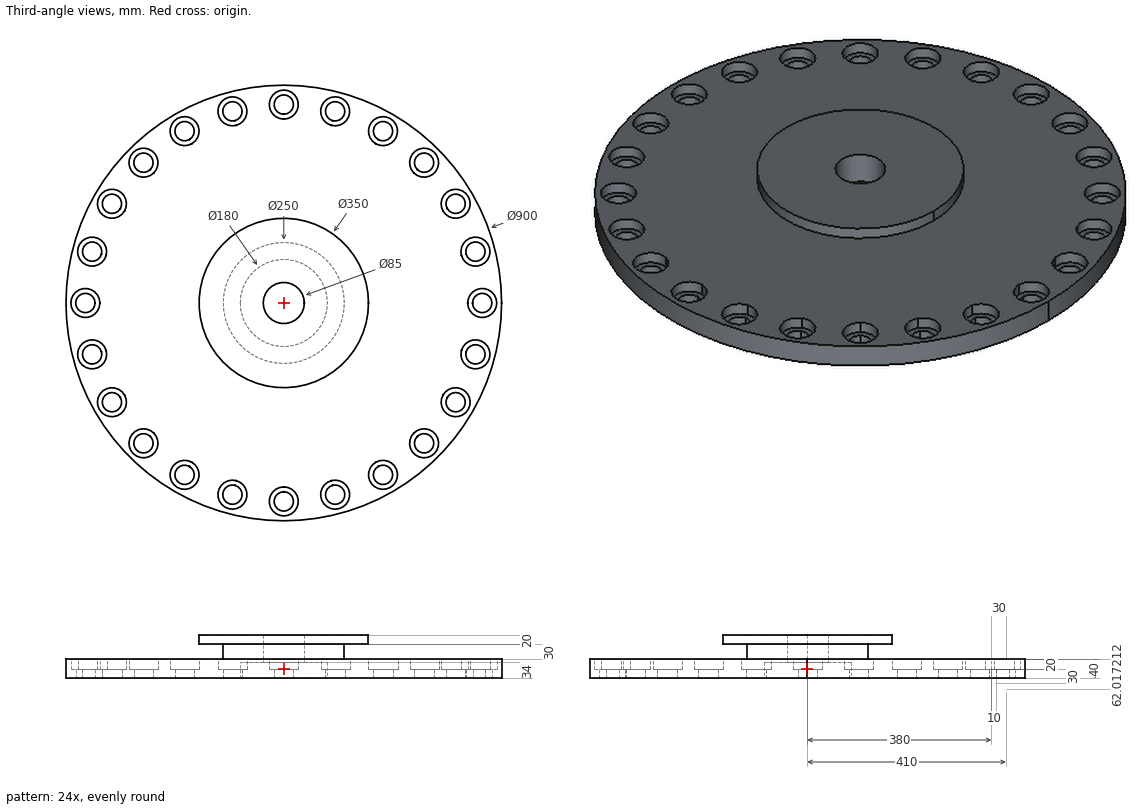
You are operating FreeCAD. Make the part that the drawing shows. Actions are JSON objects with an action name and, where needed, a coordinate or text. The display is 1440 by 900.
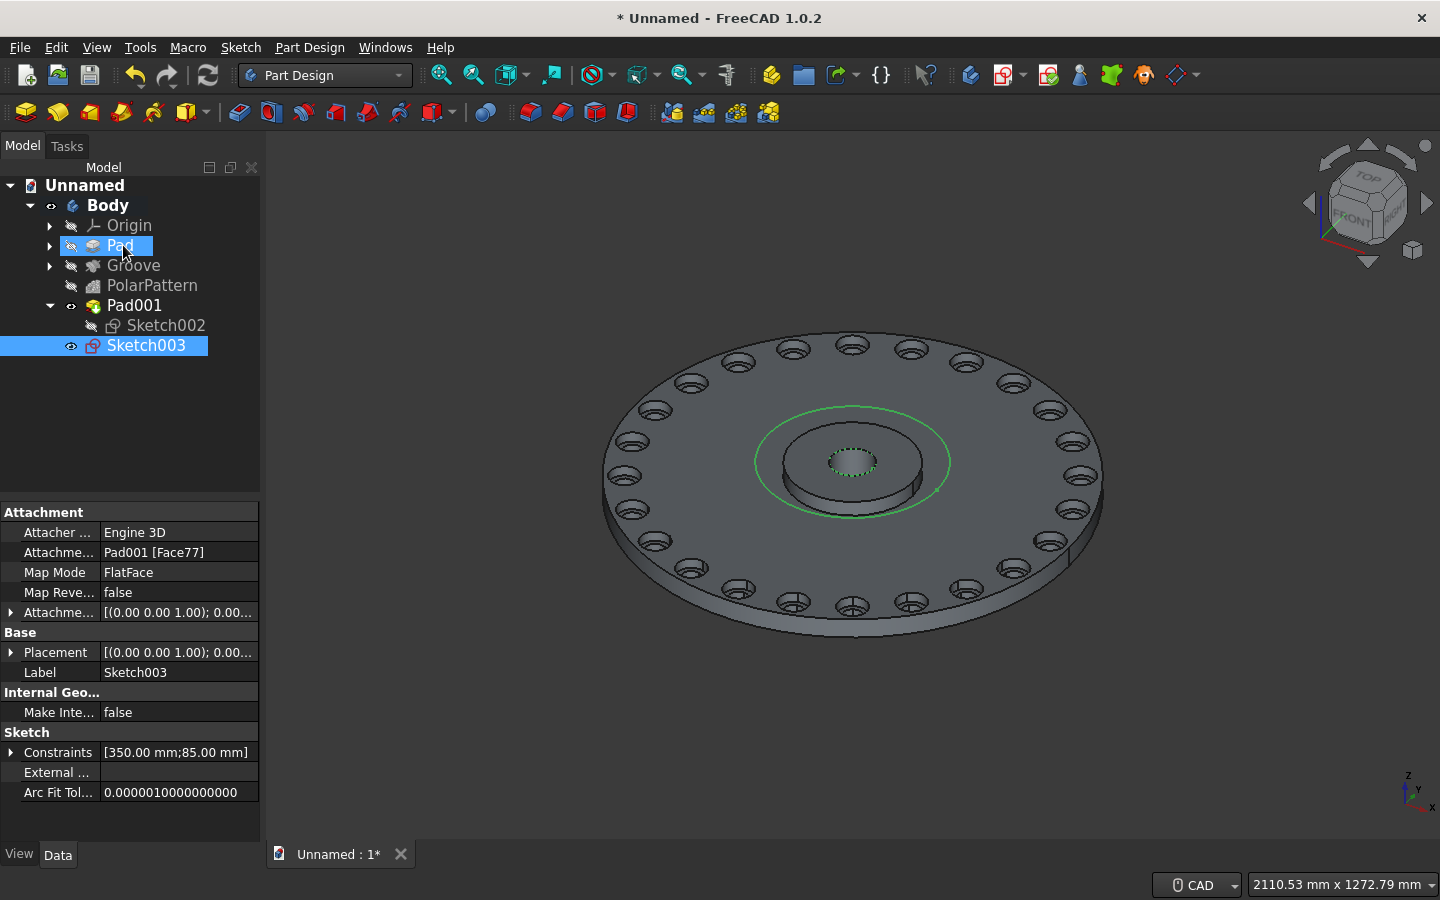
{"action": "left_click", "coordinate": [26, 112]}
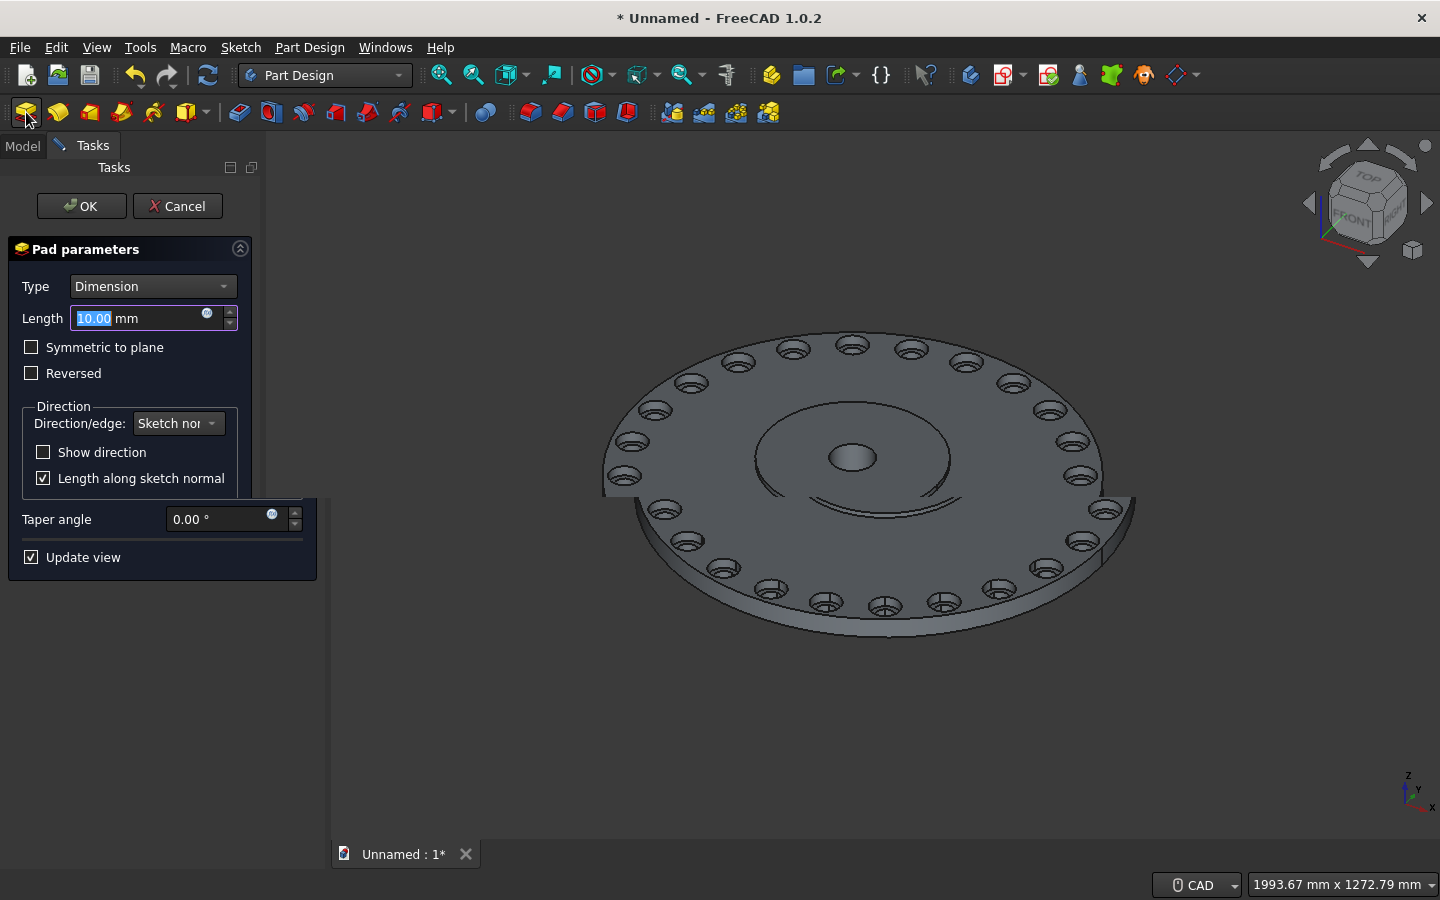
{"action": "type", "text": "20"}
{"action": "key", "text": "Tab"}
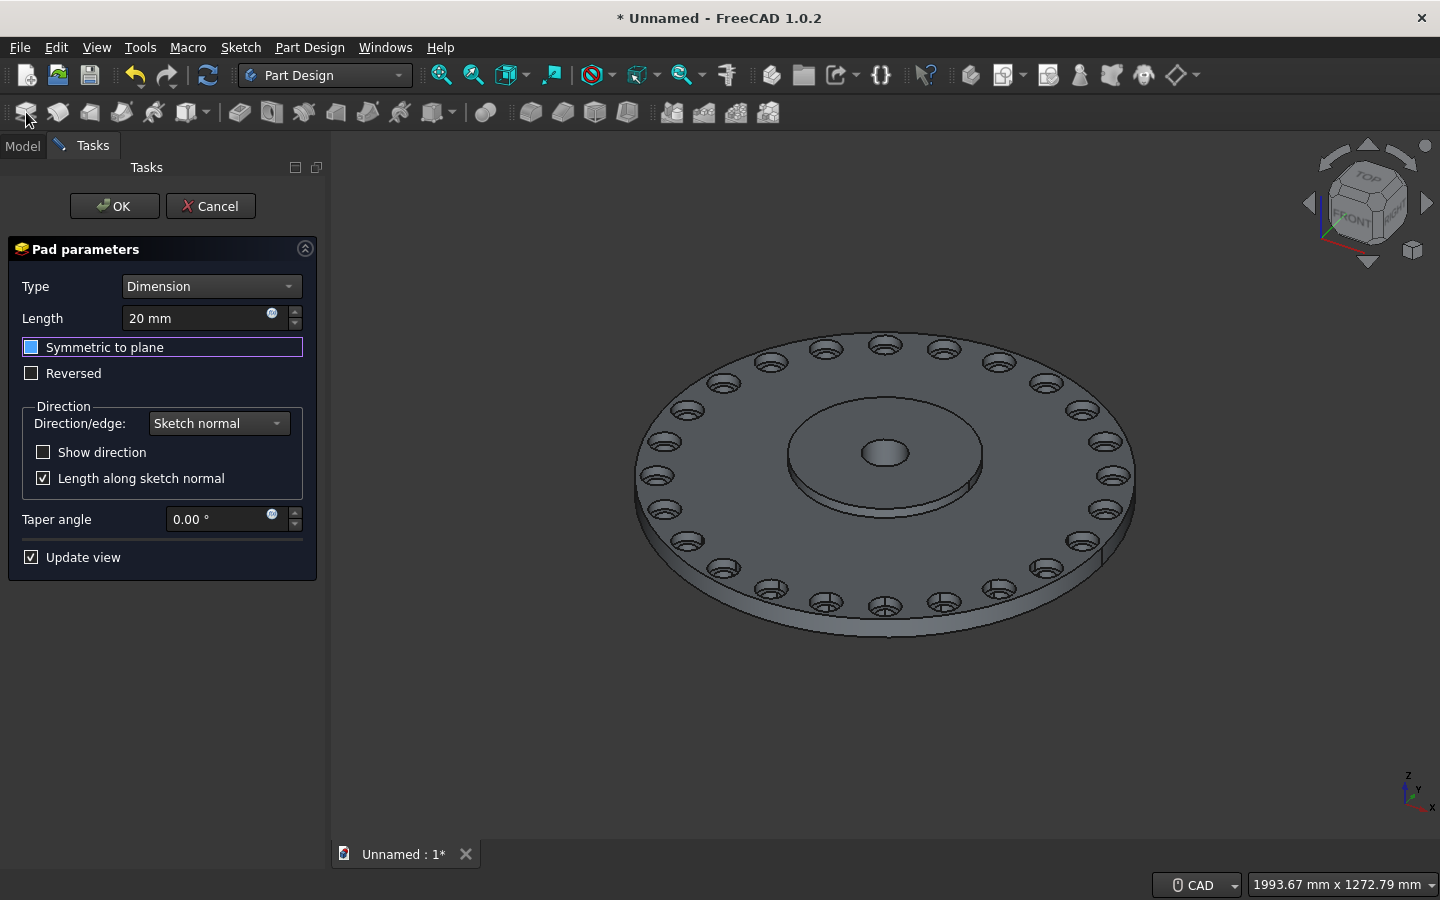
{"action": "left_click", "coordinate": [115, 206]}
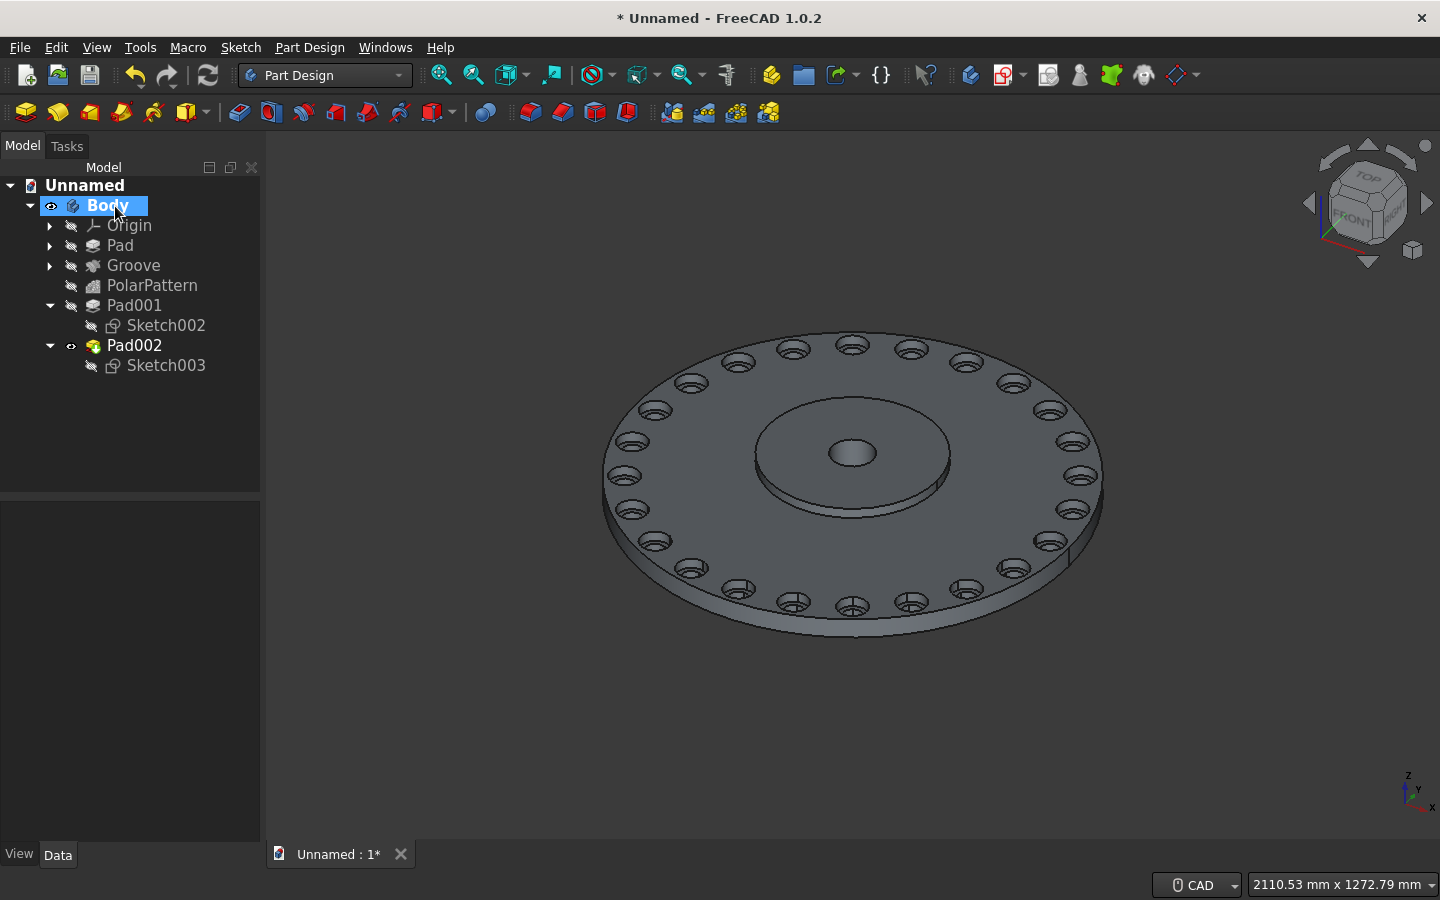
{"action": "key", "text": "5"}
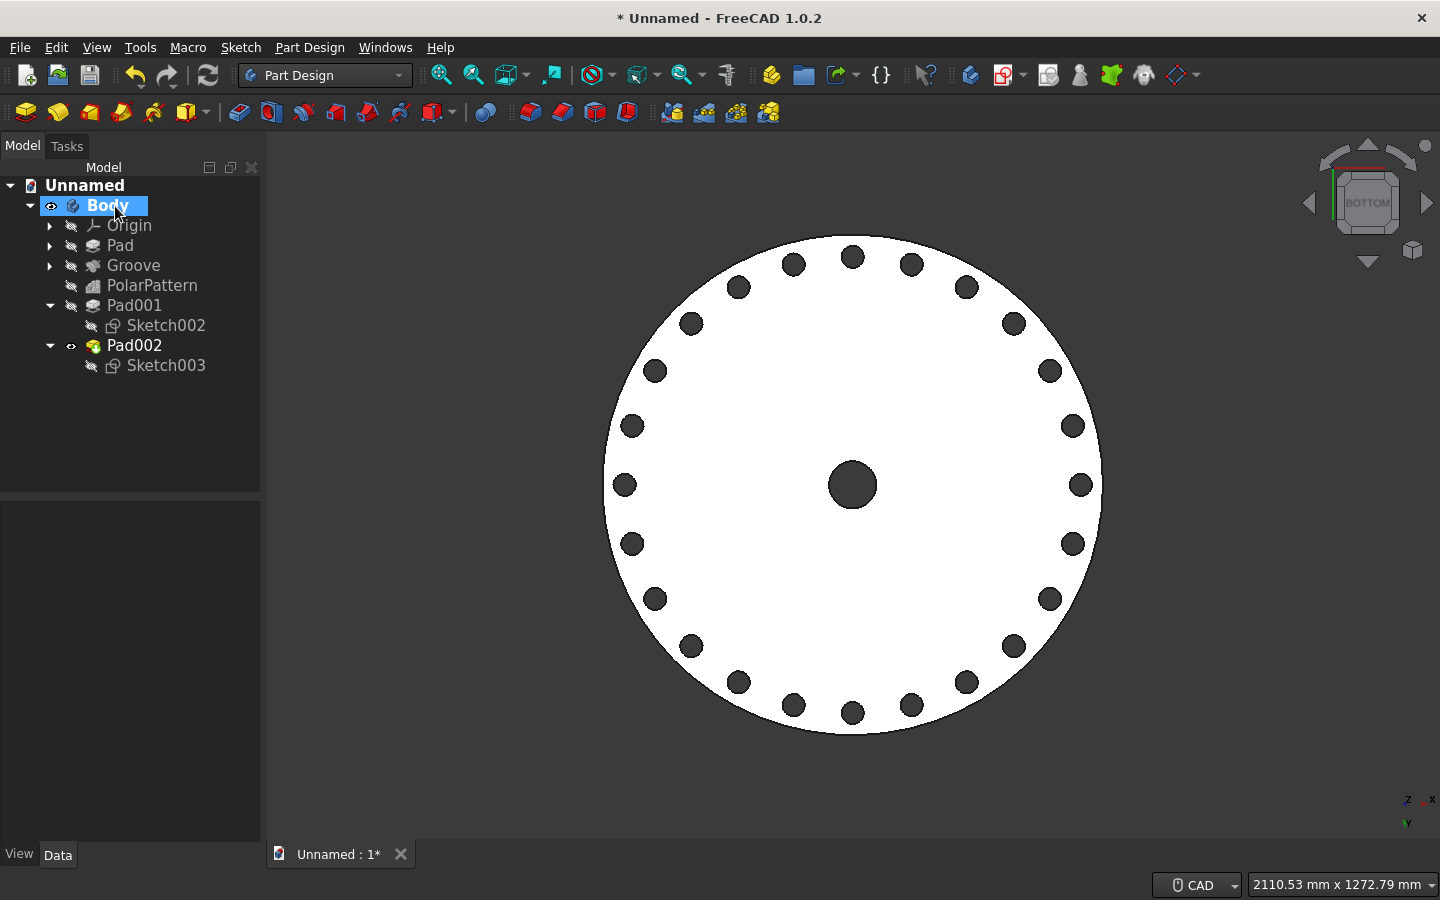
{"action": "left_click", "coordinate": [781, 412]}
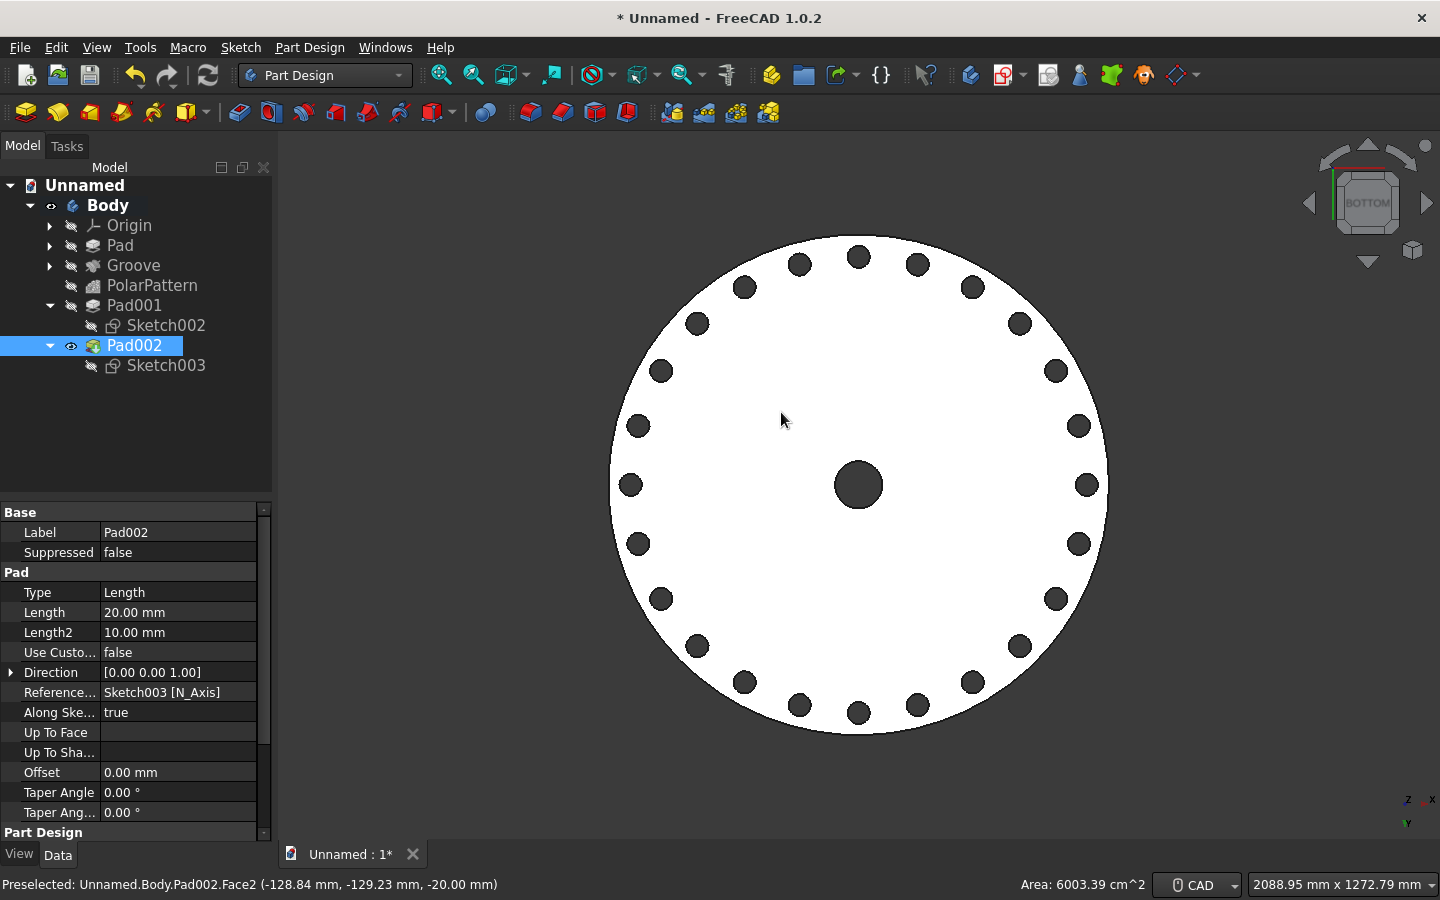
{"action": "left_click", "coordinate": [1004, 76]}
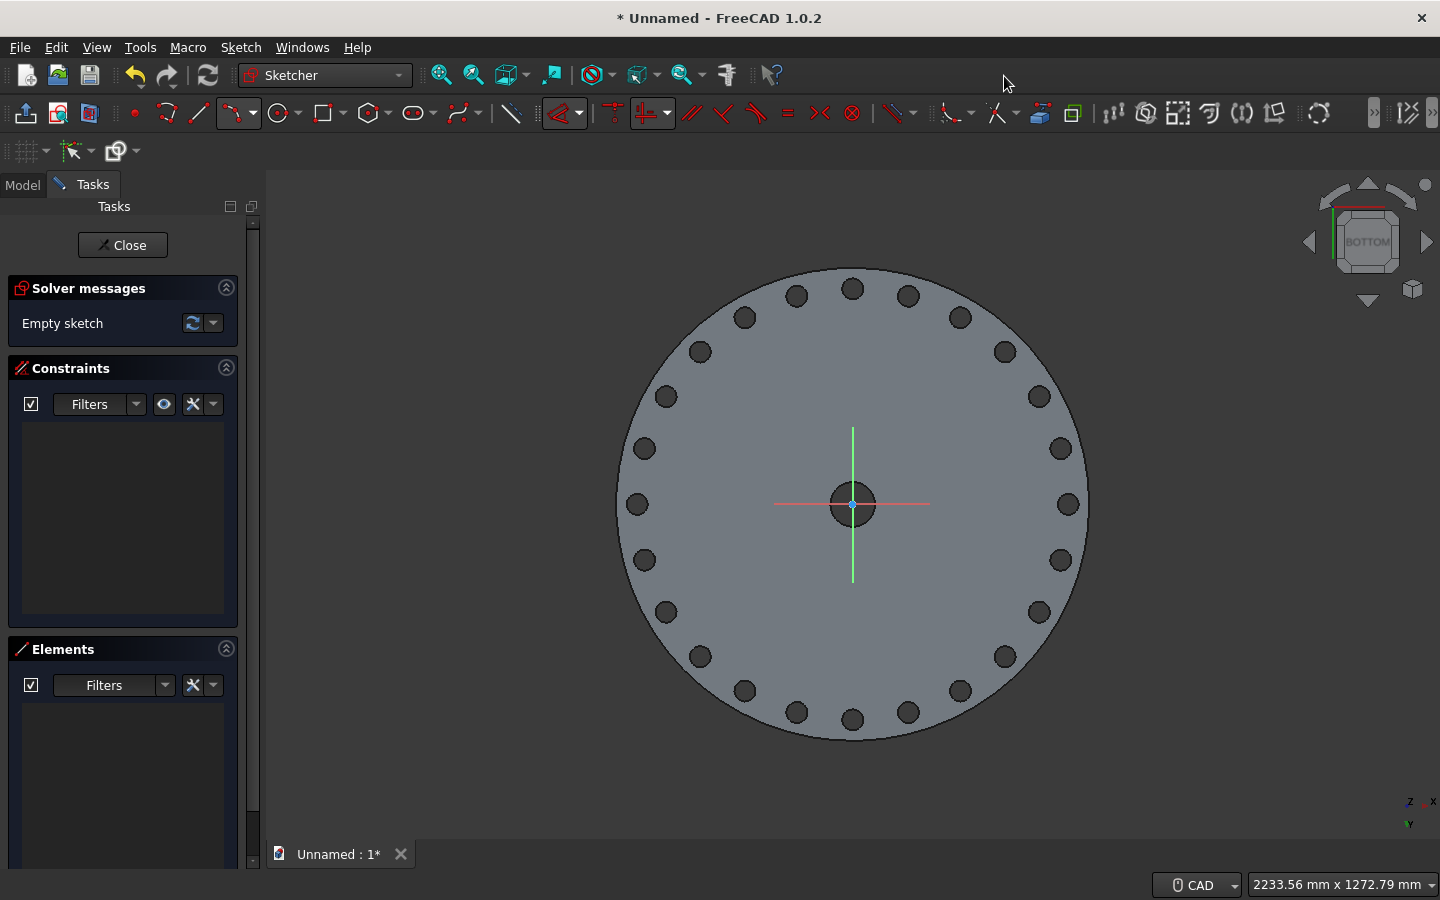
{"action": "scroll", "coordinate": [870, 504], "scroll_direction": "up", "scroll_amount": 8}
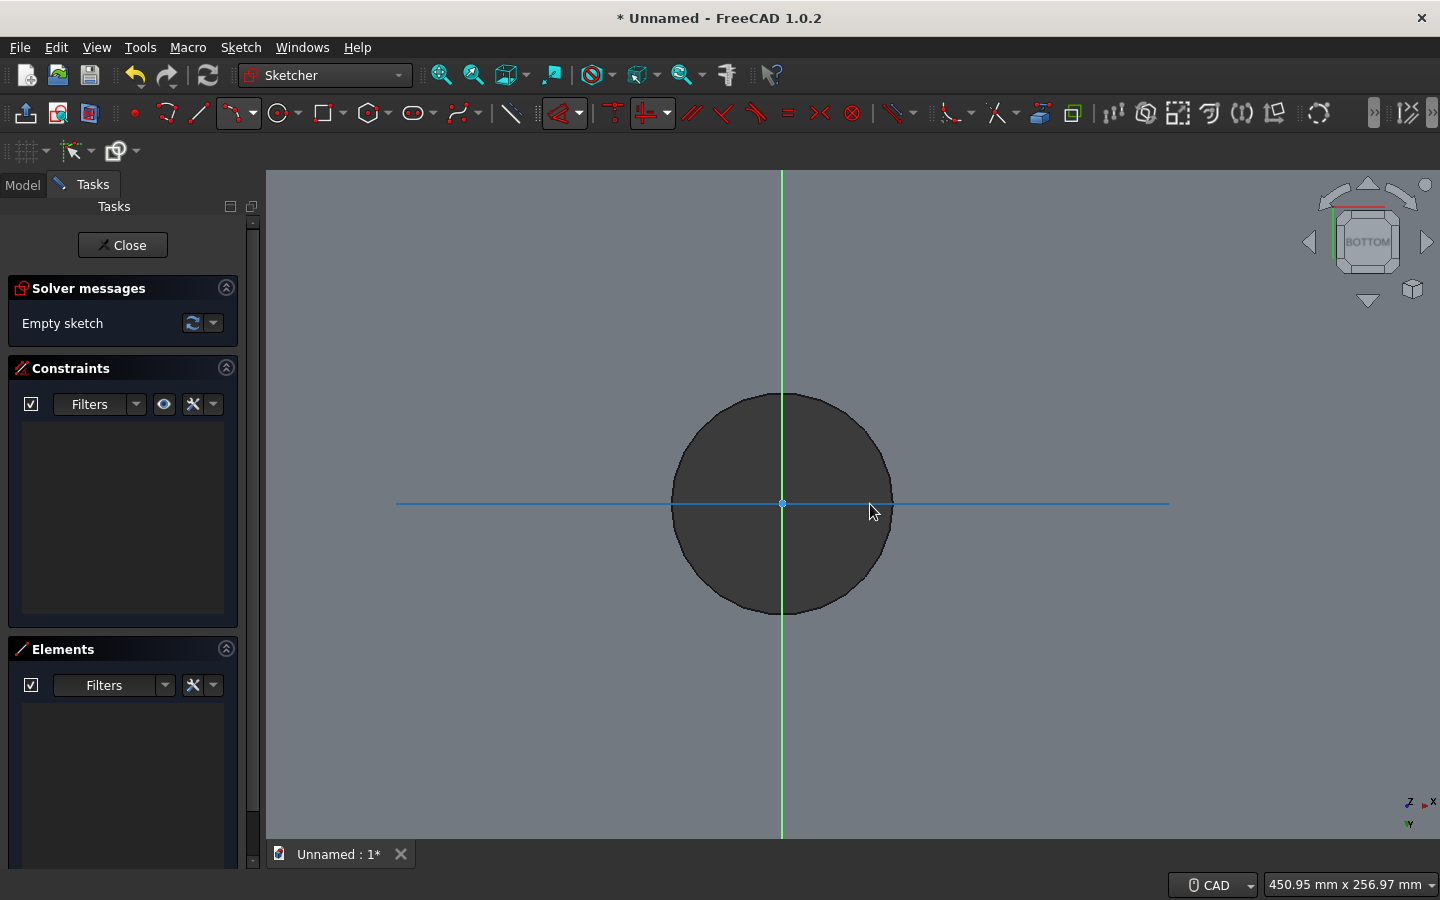
{"action": "key", "text": "g c"}